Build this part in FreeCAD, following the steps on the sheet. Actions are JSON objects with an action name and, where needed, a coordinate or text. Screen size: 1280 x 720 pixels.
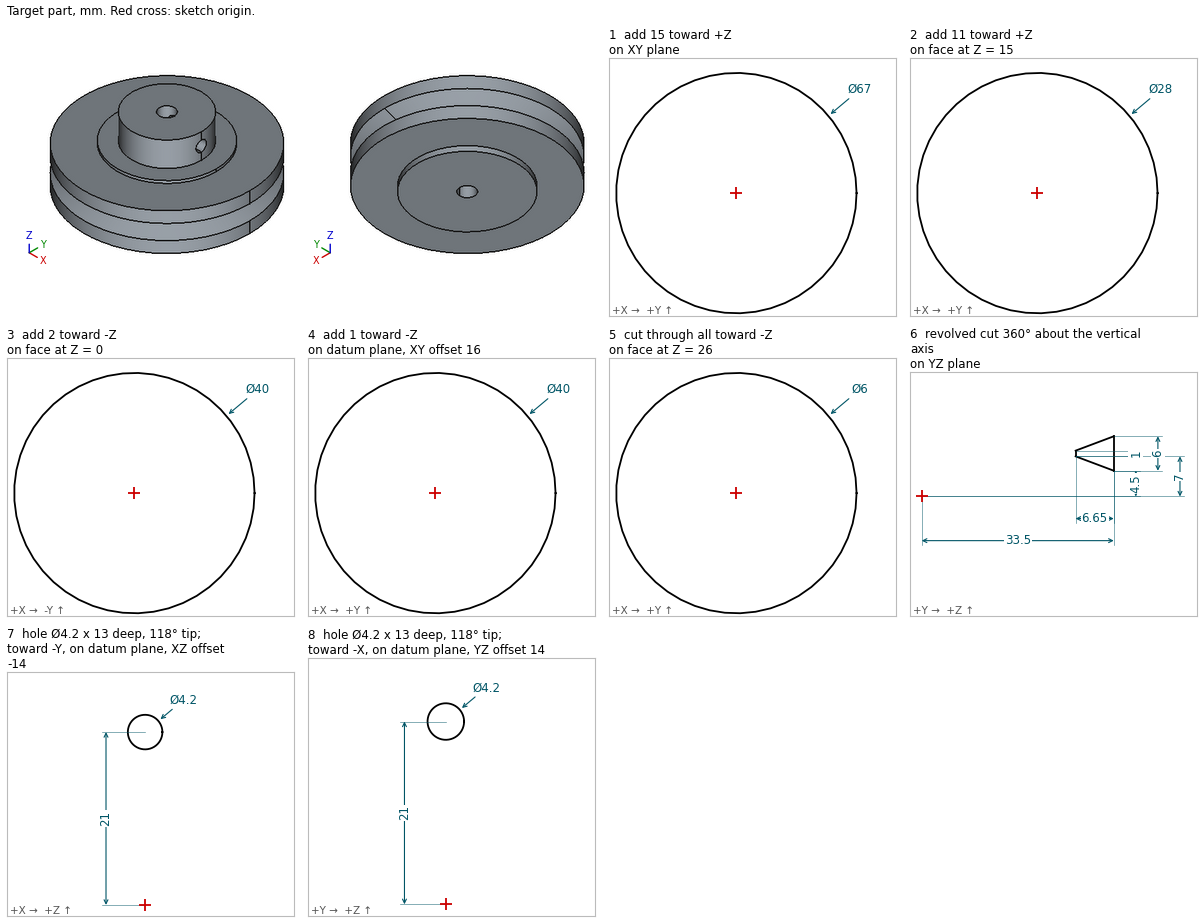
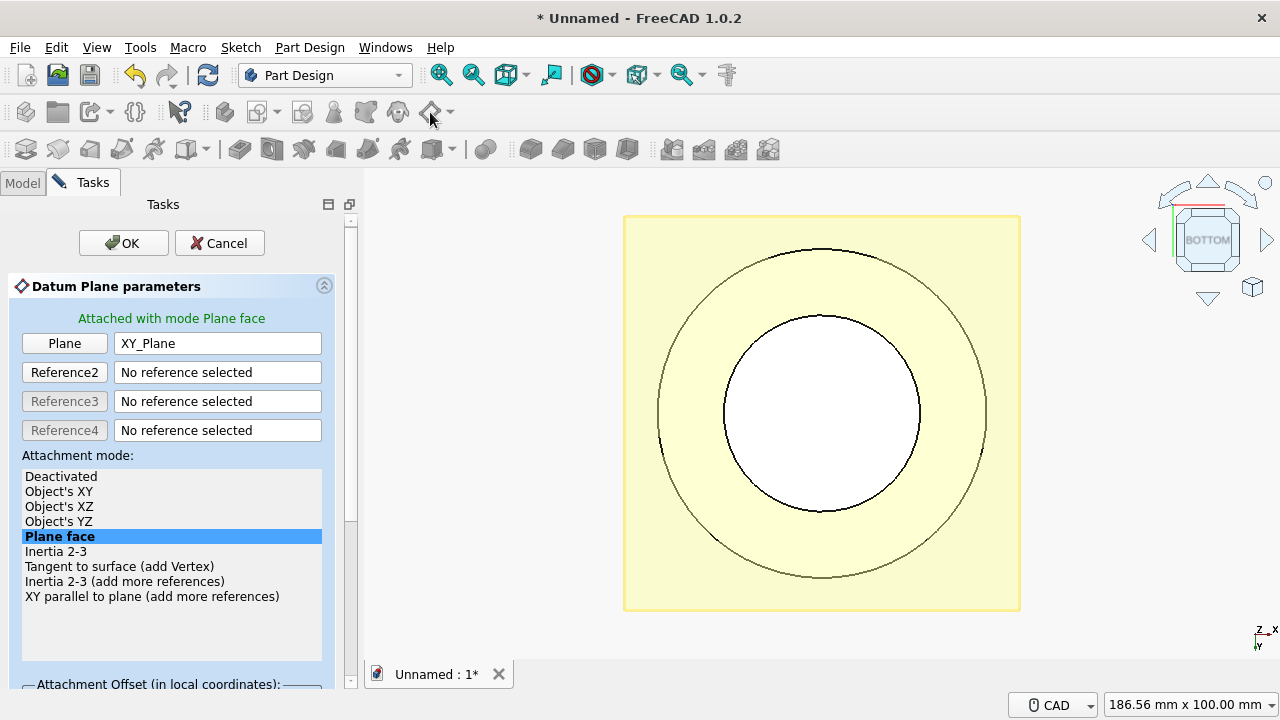
{"action": "scroll", "coordinate": [351, 451], "scroll_direction": "down", "scroll_amount": 3}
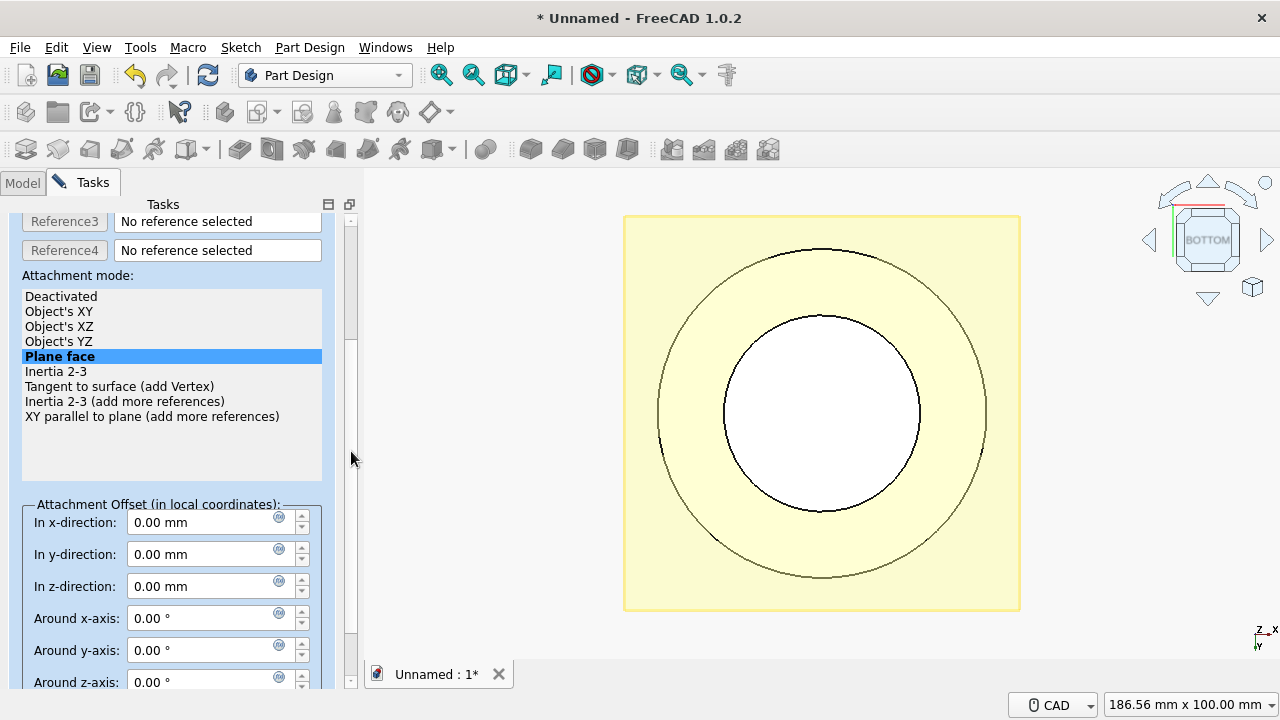
{"action": "triple_click", "coordinate": [210, 586]}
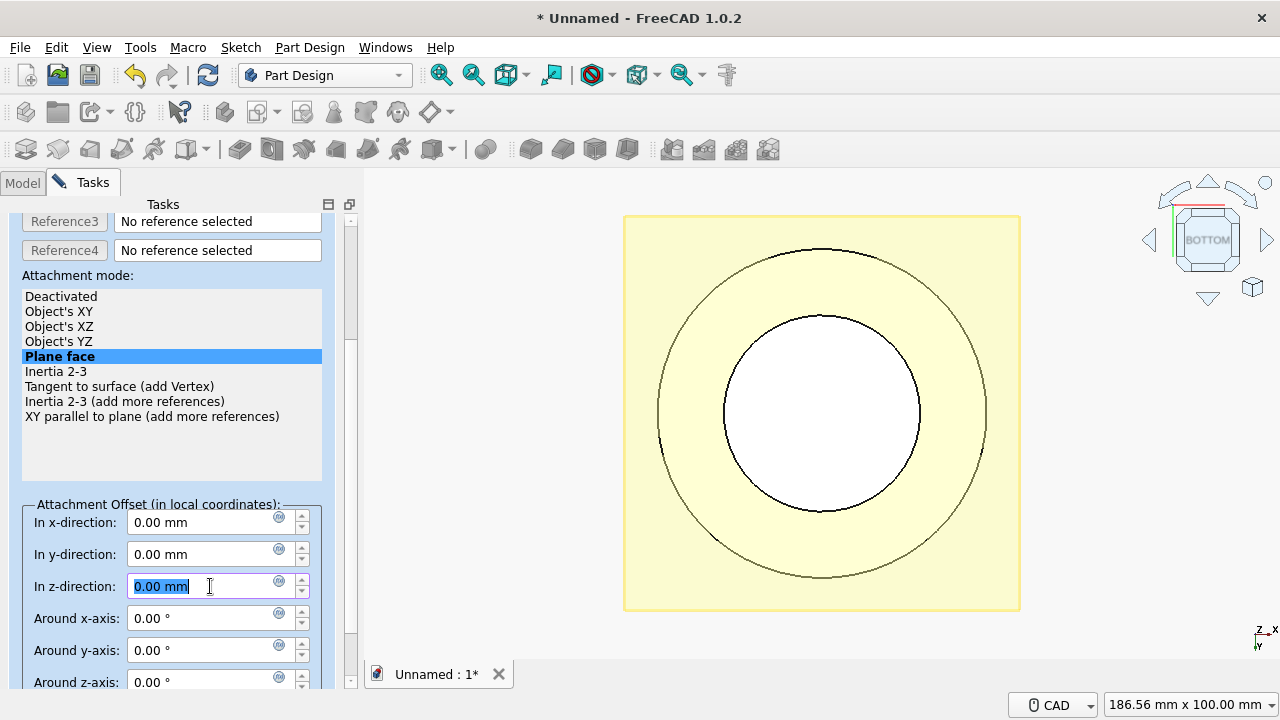
{"action": "type", "text": "16"}
{"action": "key", "text": "Tab"}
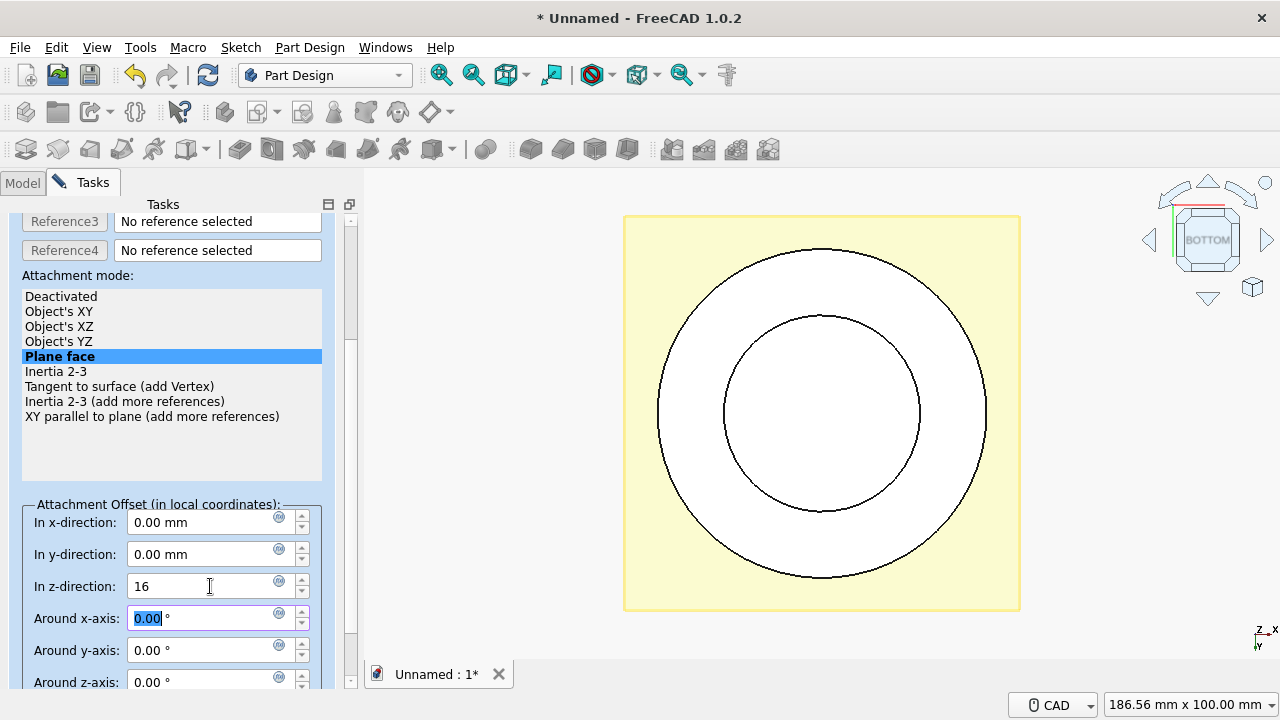
{"action": "scroll", "coordinate": [351, 451], "scroll_direction": "up", "scroll_amount": 4}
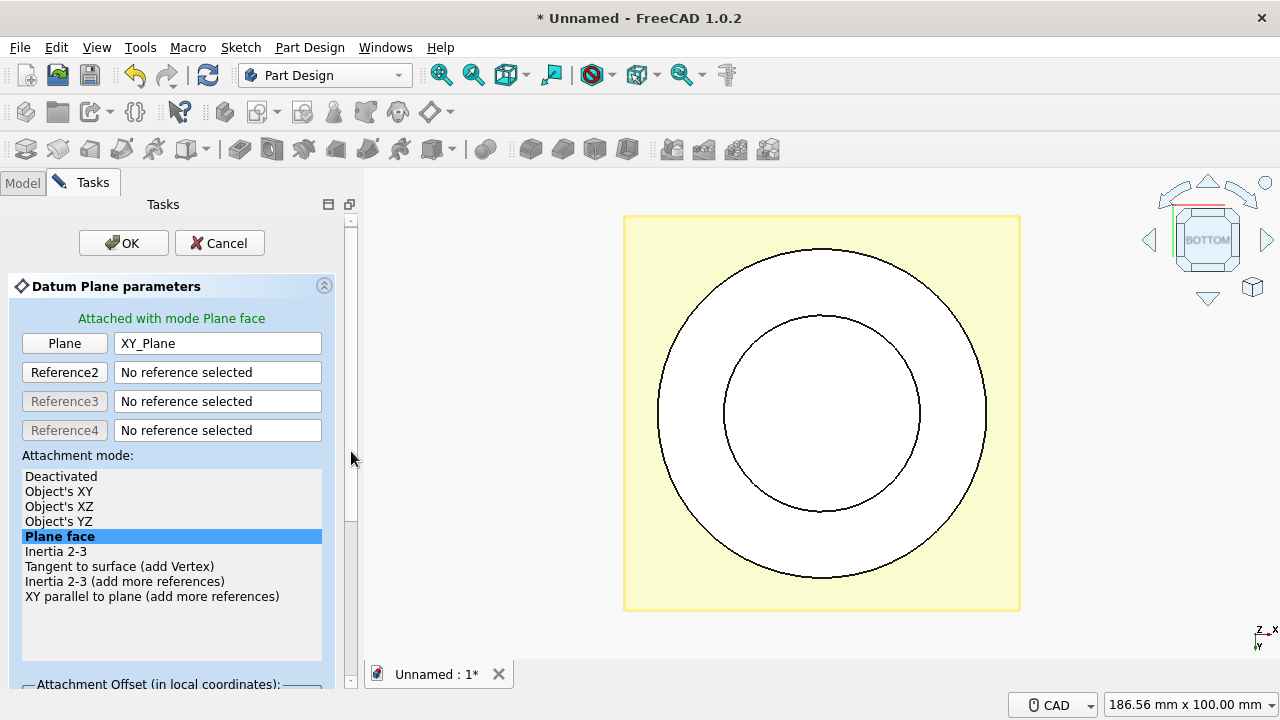
{"action": "left_click", "coordinate": [124, 243]}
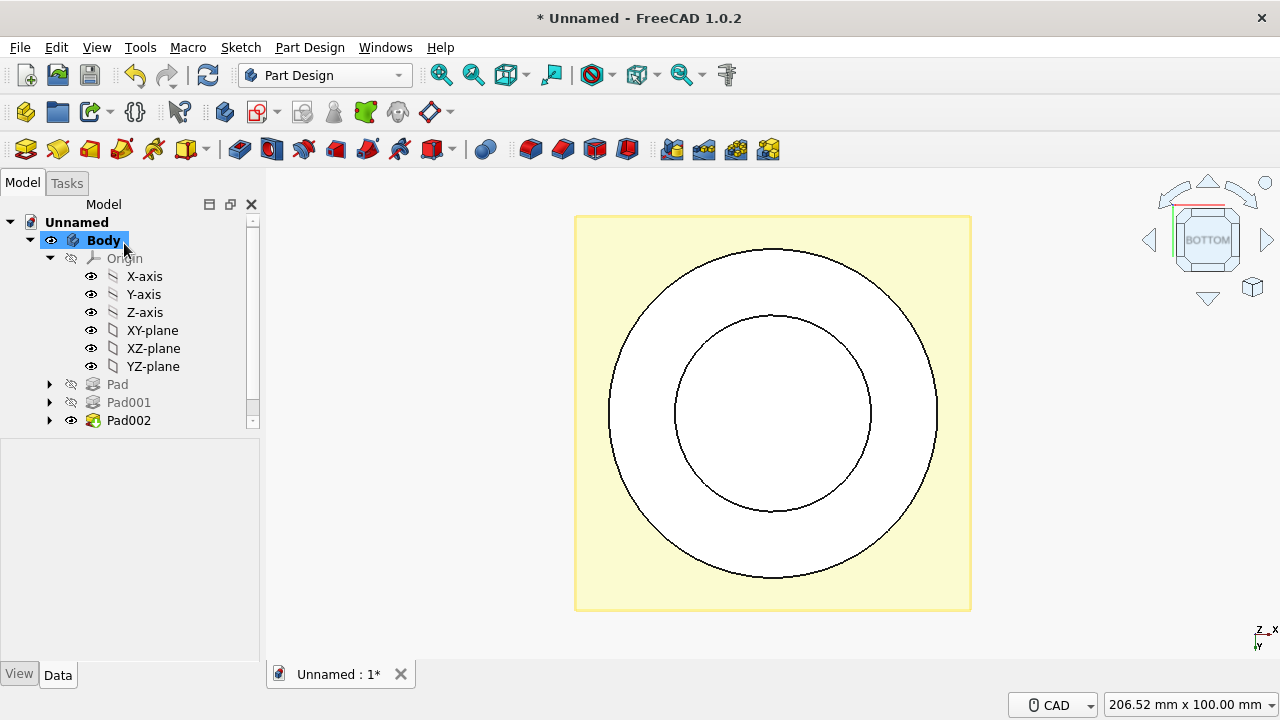
{"action": "scroll", "coordinate": [100, 326], "scroll_direction": "down", "scroll_amount": 3}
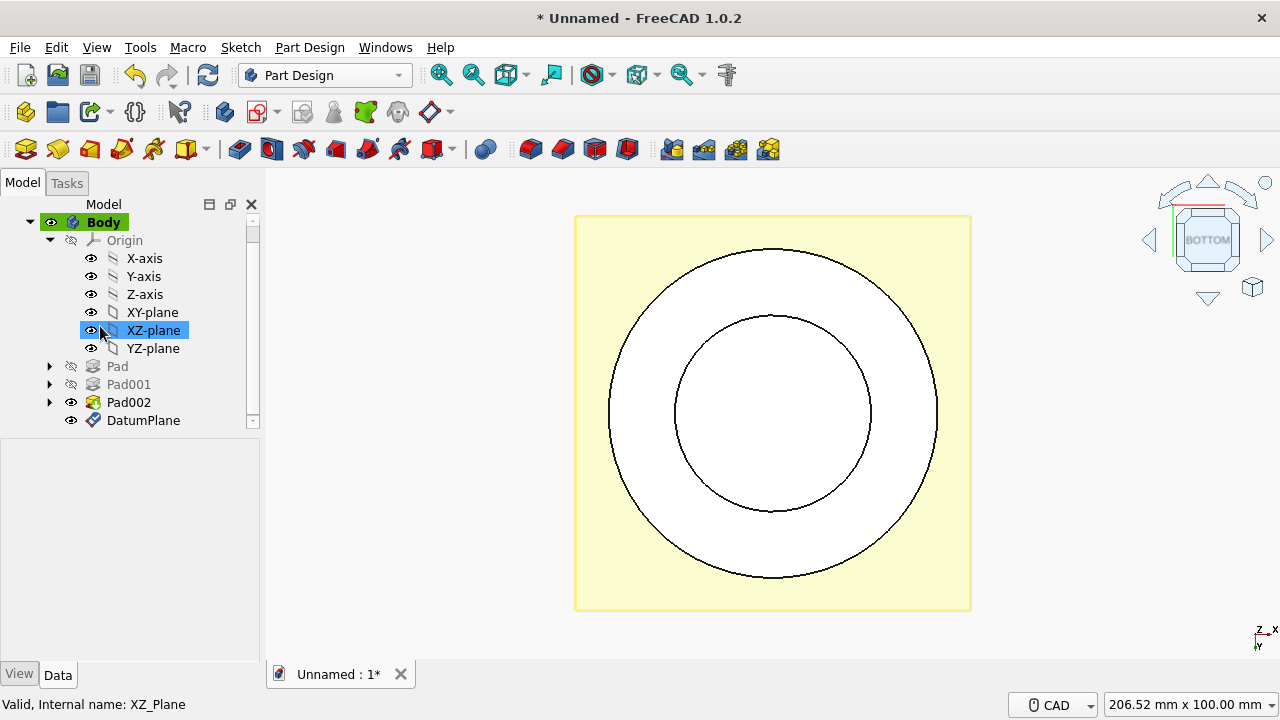
{"action": "left_click", "coordinate": [116, 420]}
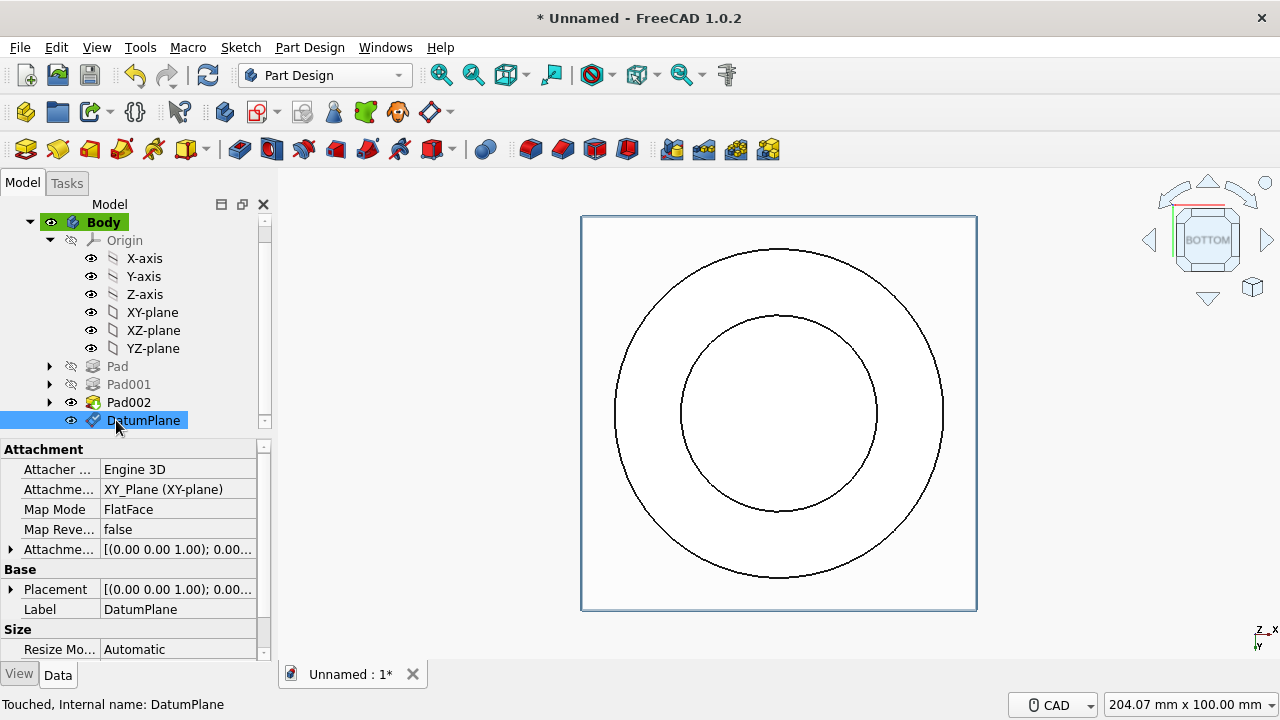
{"action": "left_click", "coordinate": [258, 112]}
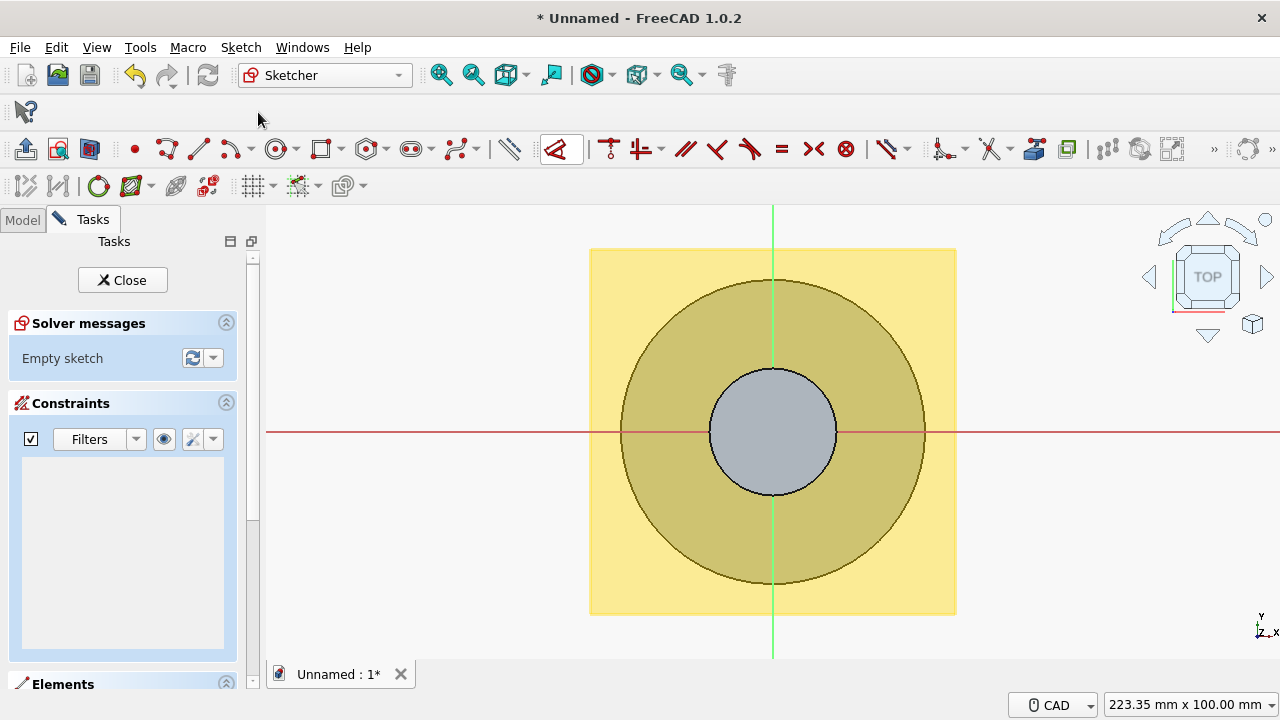
{"action": "left_click", "coordinate": [90, 150]}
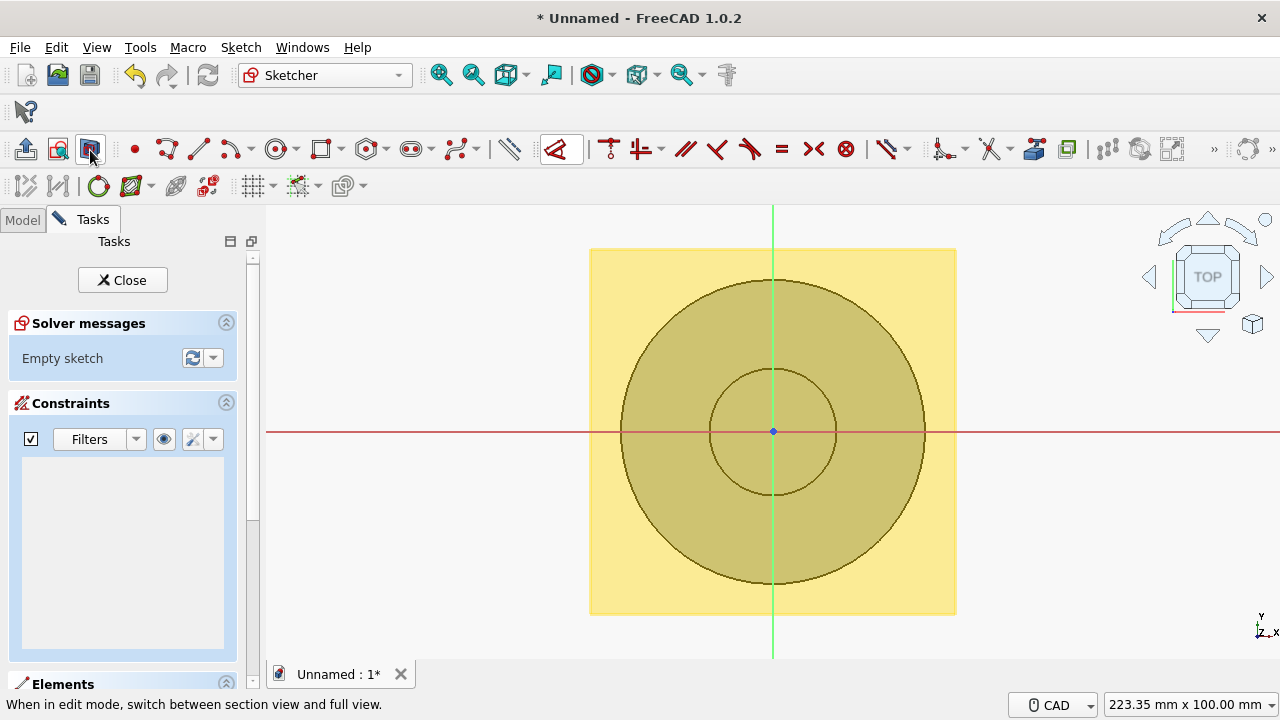
{"action": "scroll", "coordinate": [912, 432], "scroll_direction": "up", "scroll_amount": 2}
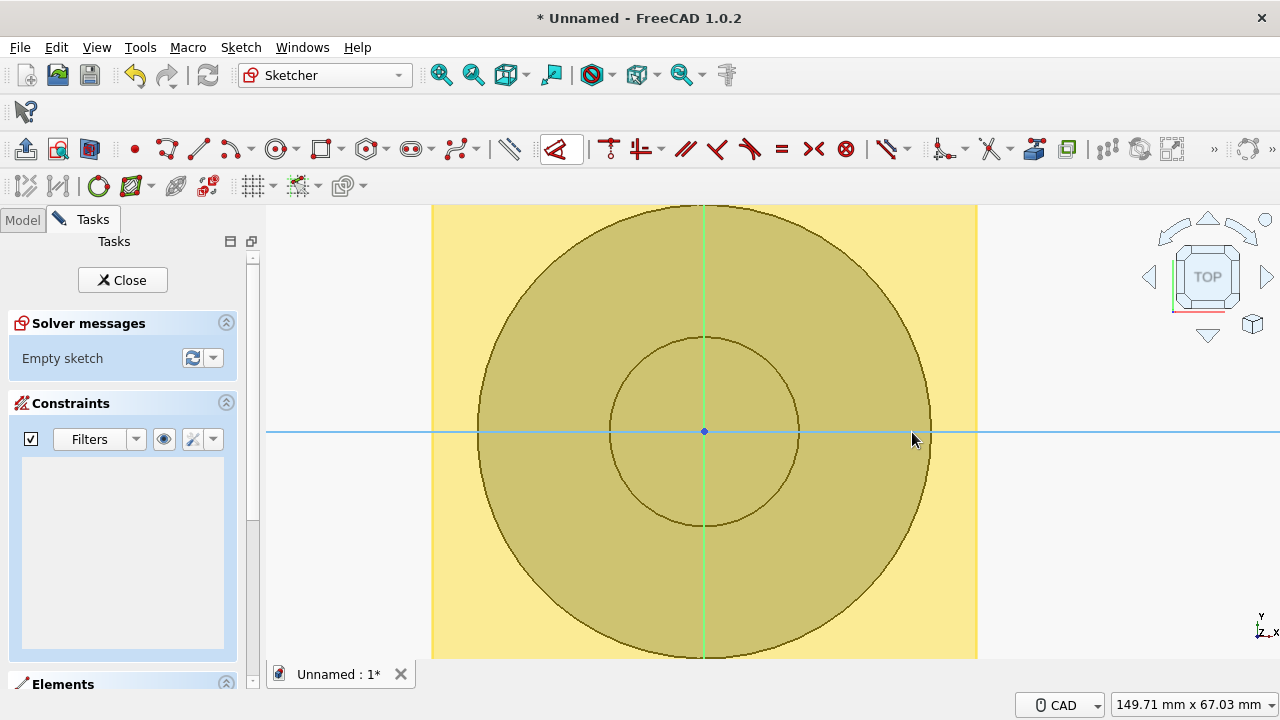
{"action": "key", "text": "g c"}